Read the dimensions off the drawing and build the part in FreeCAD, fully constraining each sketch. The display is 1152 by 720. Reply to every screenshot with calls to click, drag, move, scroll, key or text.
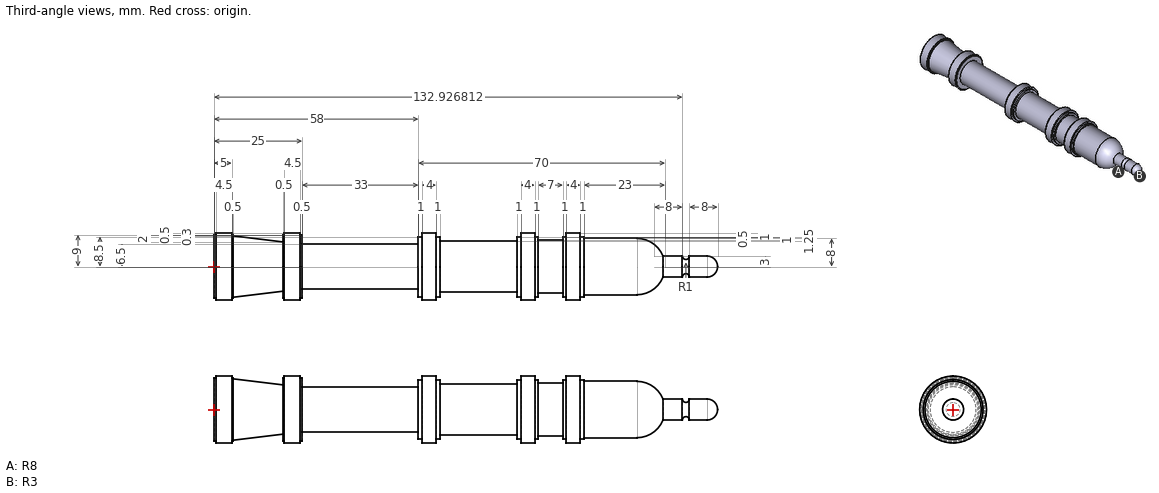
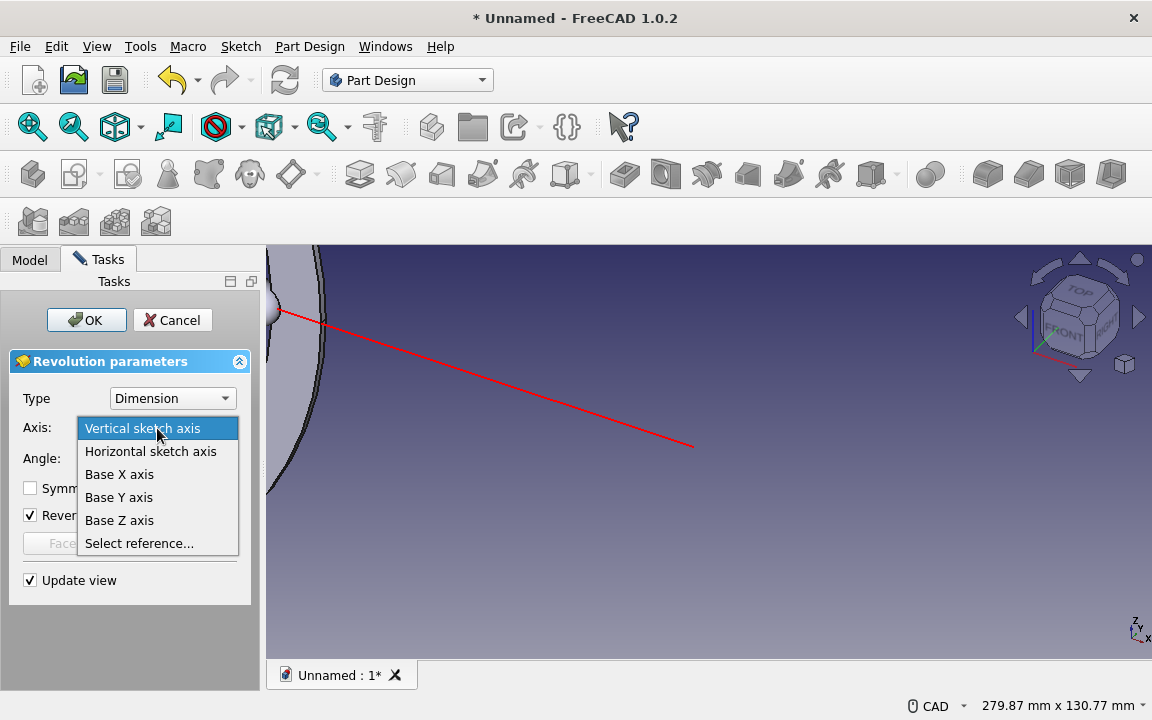
click(156, 452)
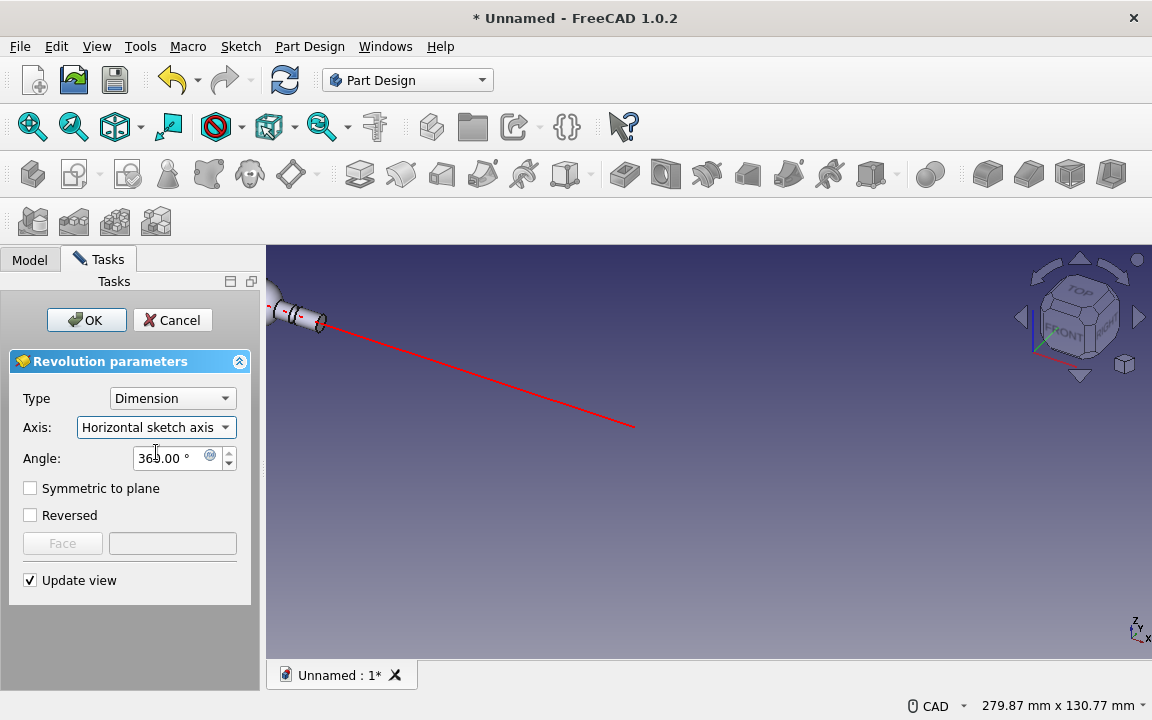
click(87, 320)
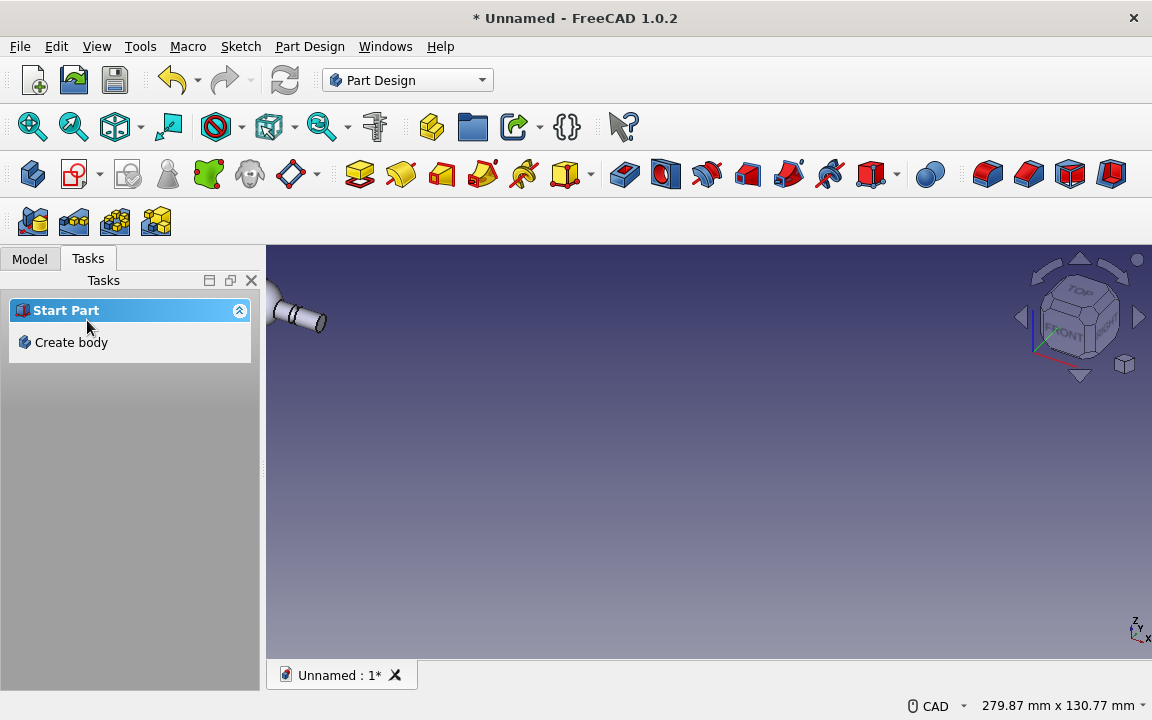
click(33, 128)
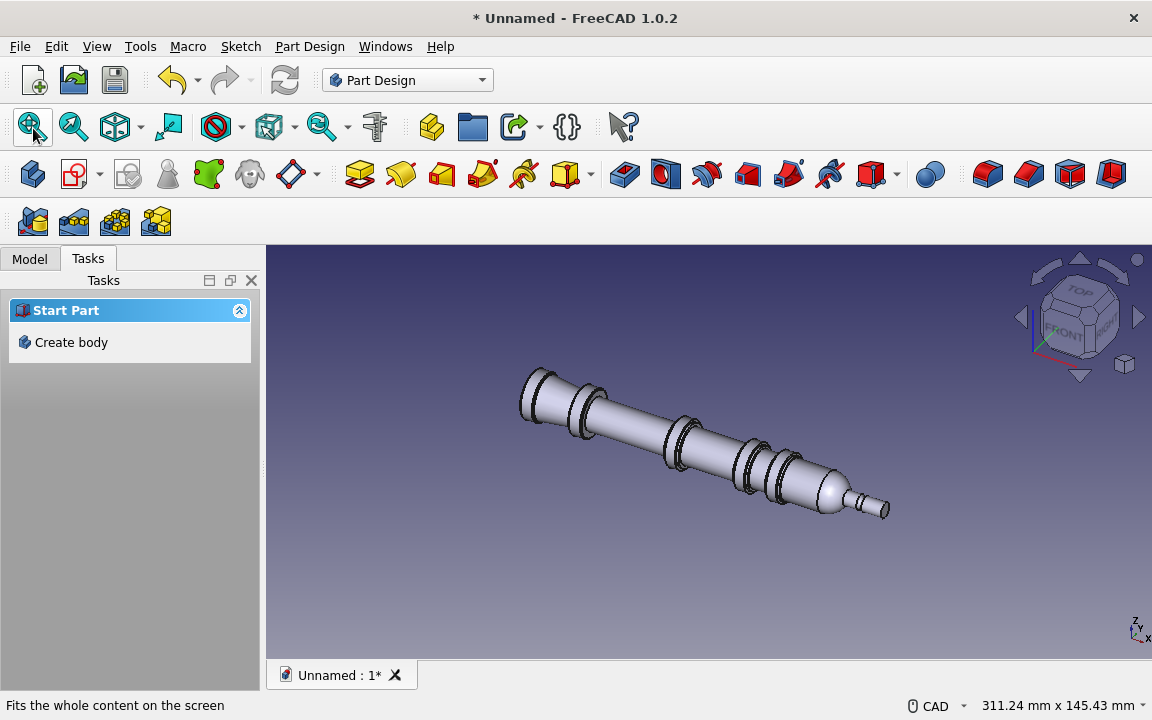
click(881, 514)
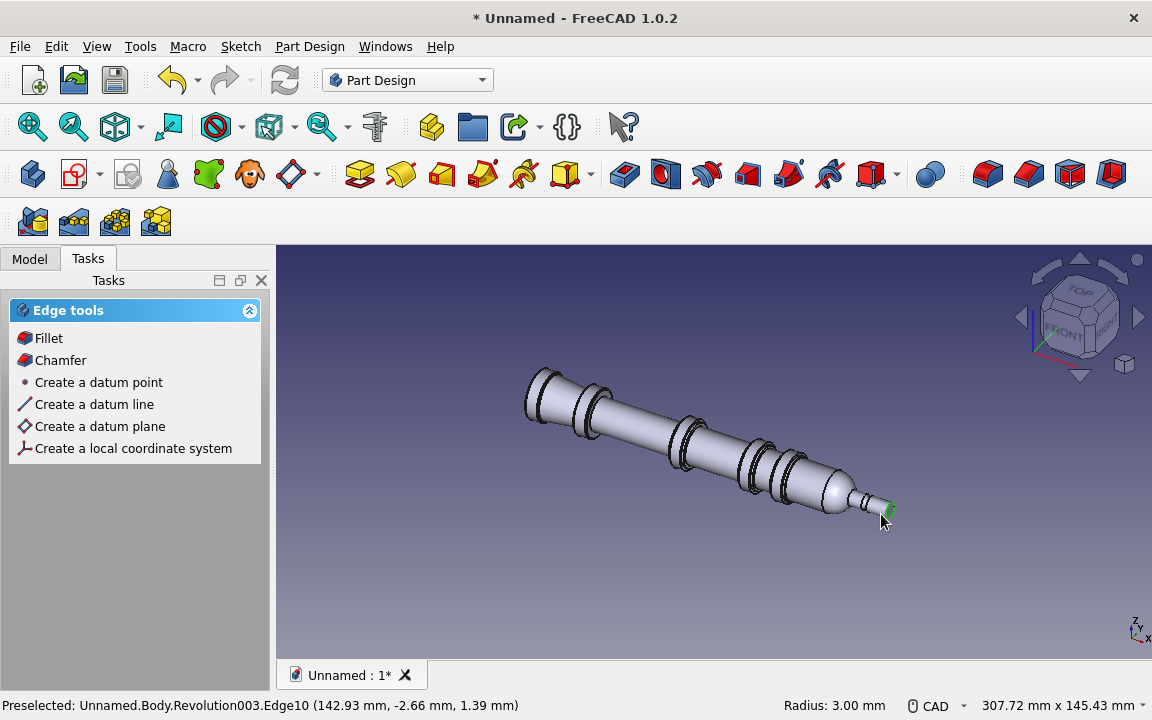
click(988, 174)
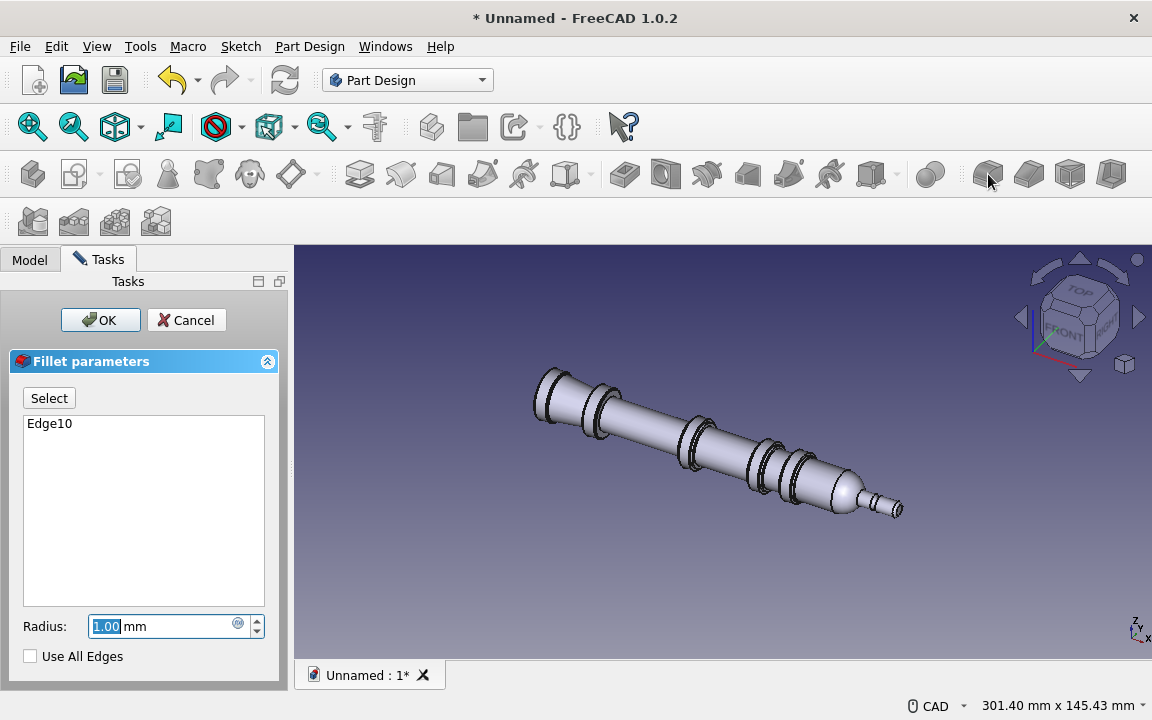
text(3)
key(Tab)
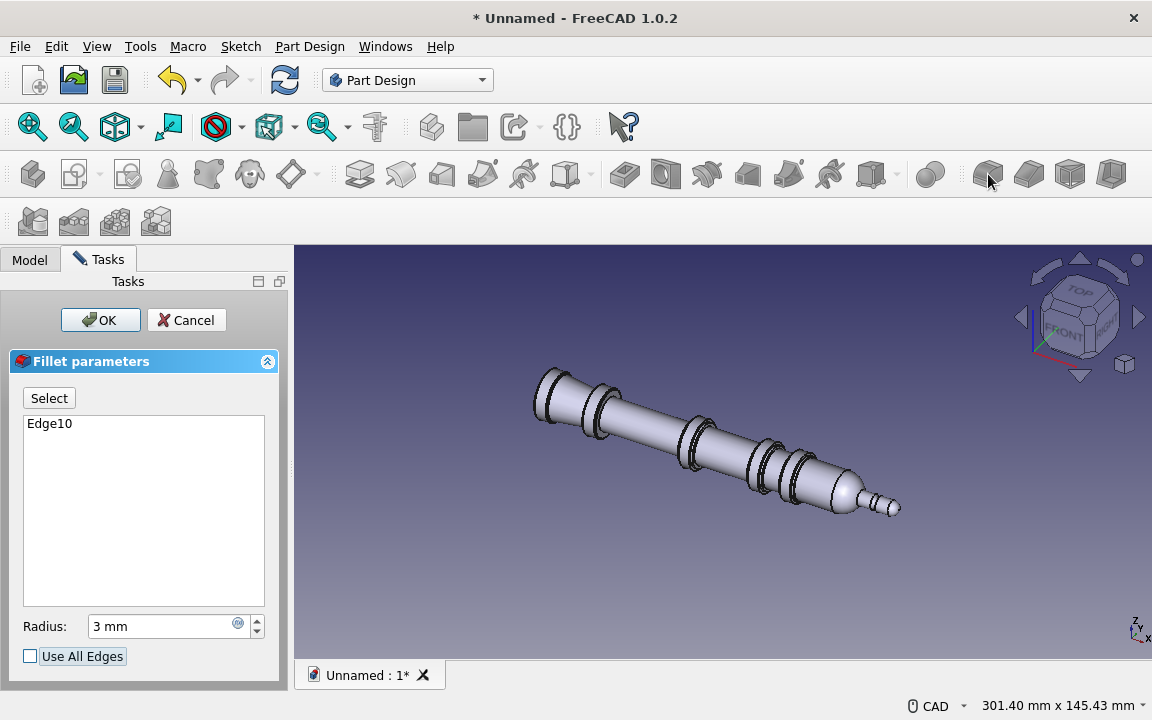
click(101, 320)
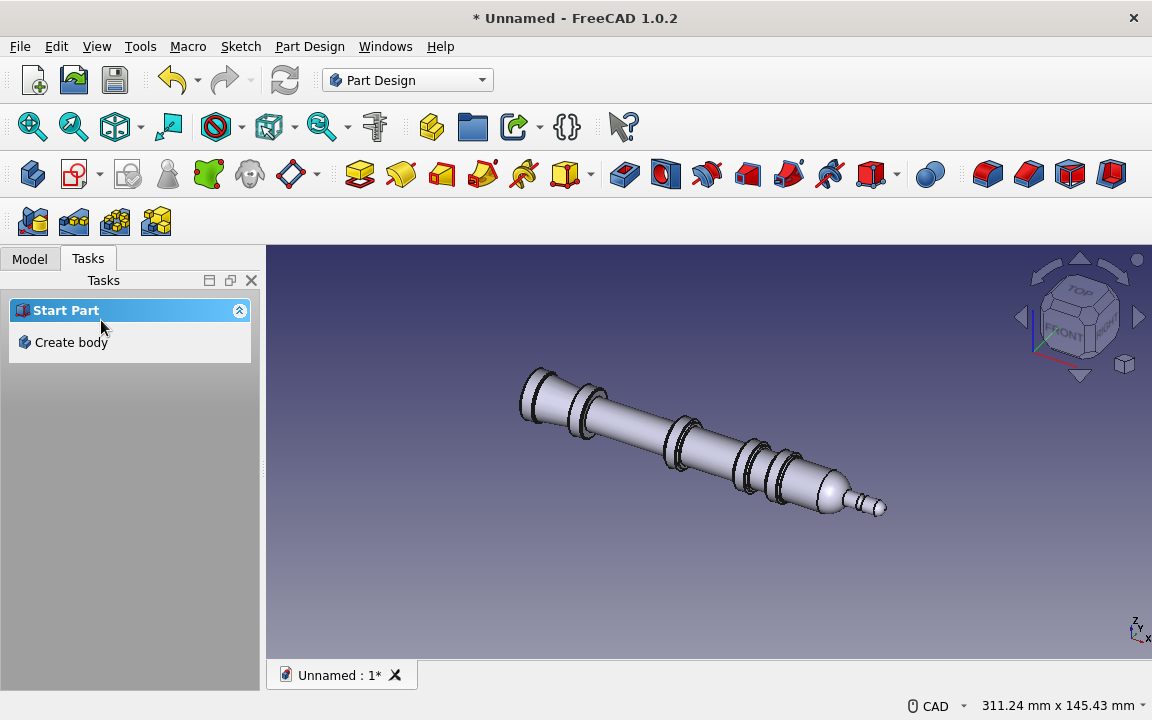
key(0)